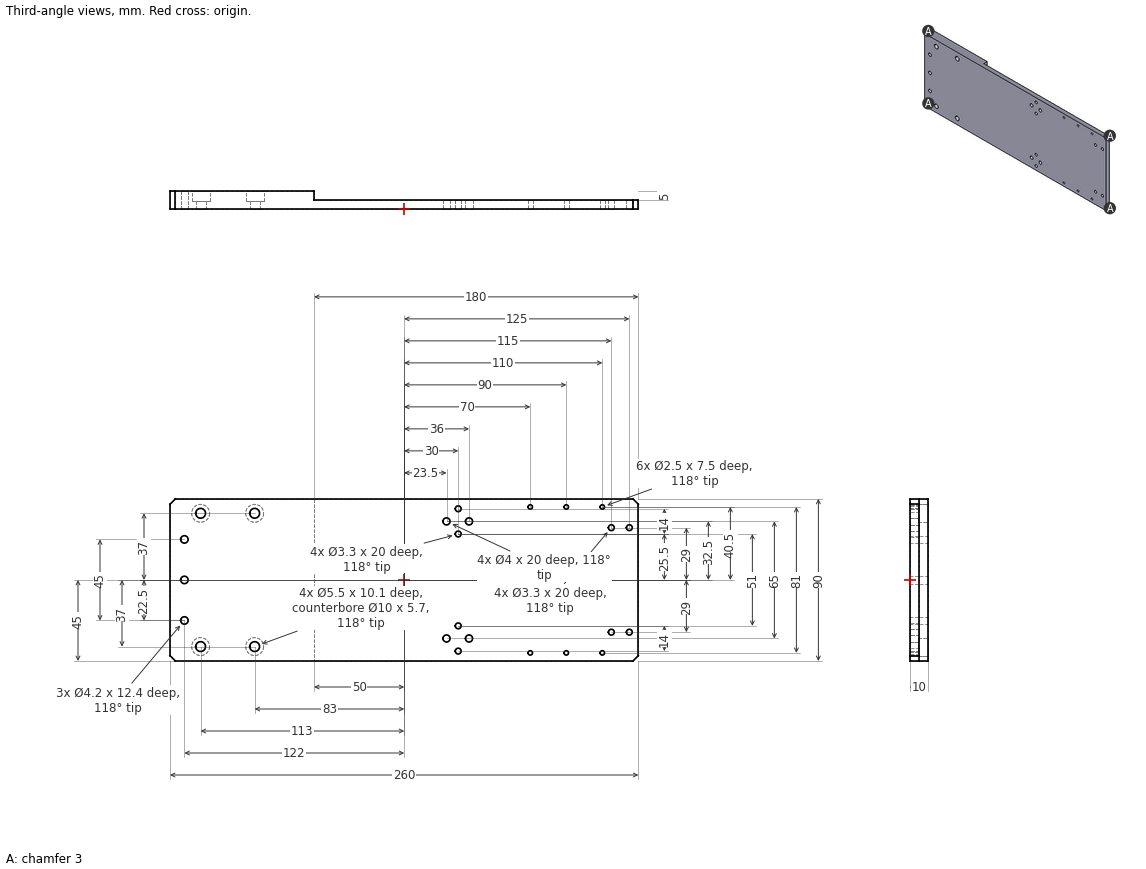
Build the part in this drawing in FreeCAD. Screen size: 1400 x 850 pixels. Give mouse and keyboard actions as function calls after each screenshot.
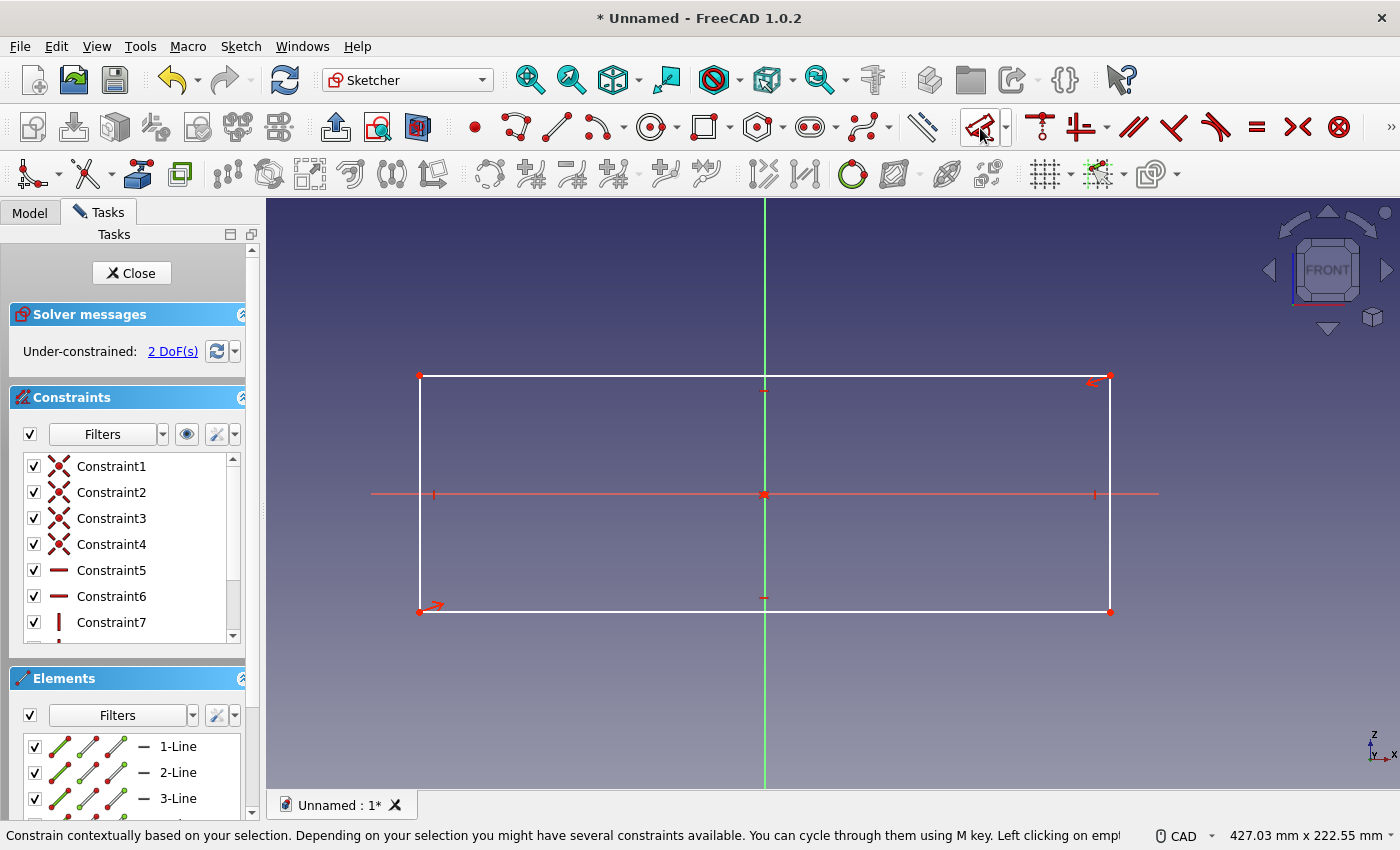
click(1110, 541)
click(1144, 440)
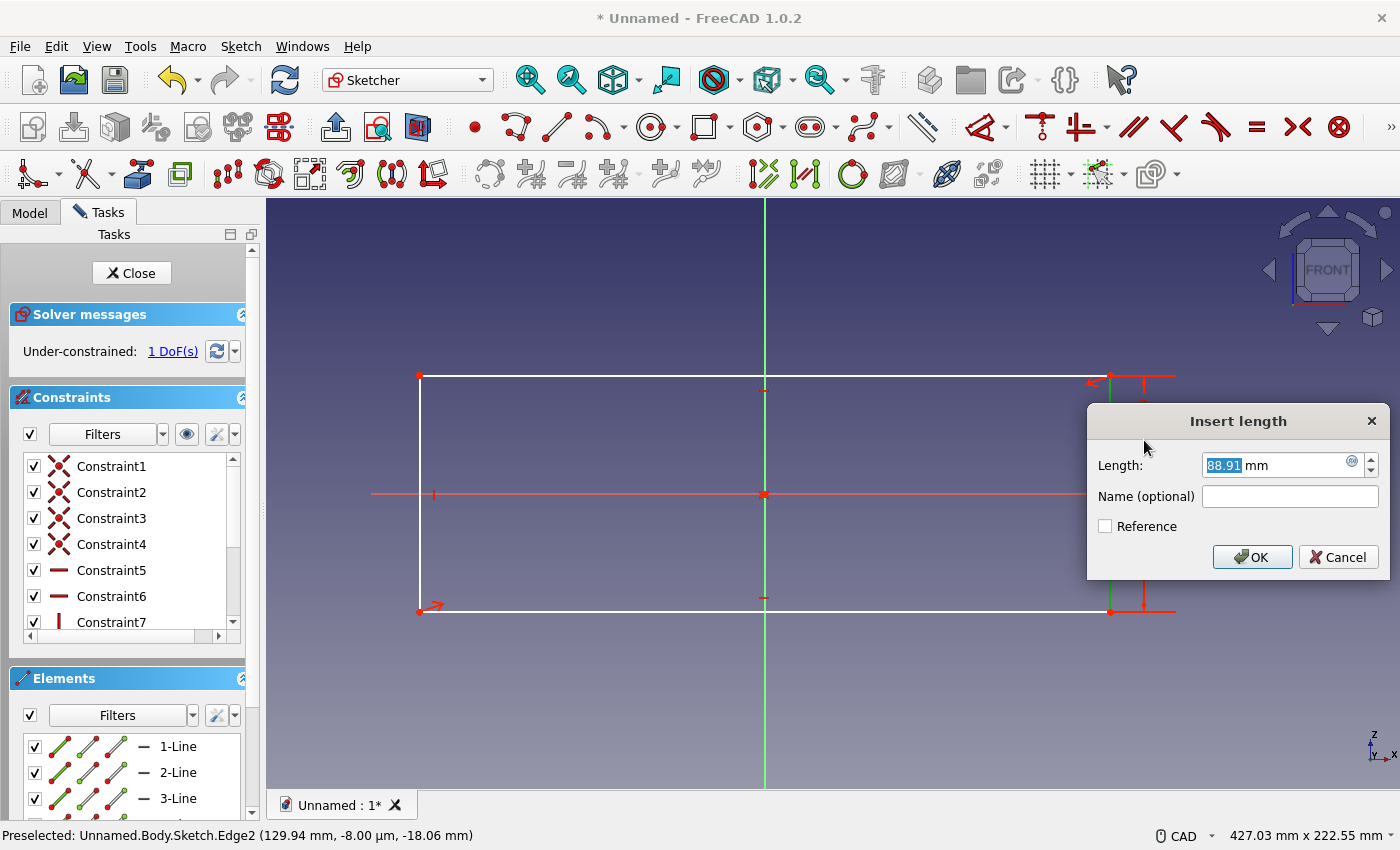
text(90)
key(Return)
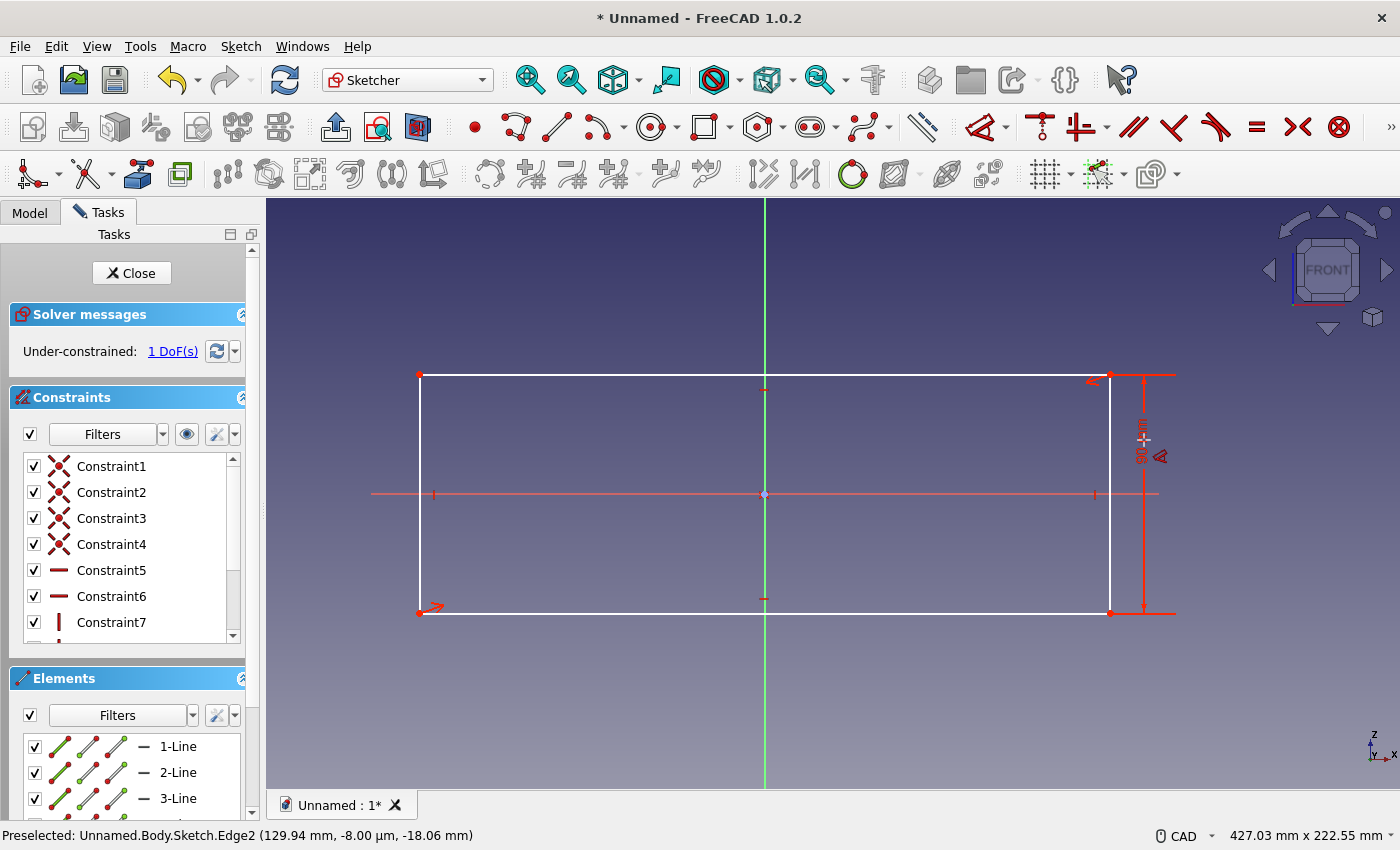
click(627, 614)
click(606, 648)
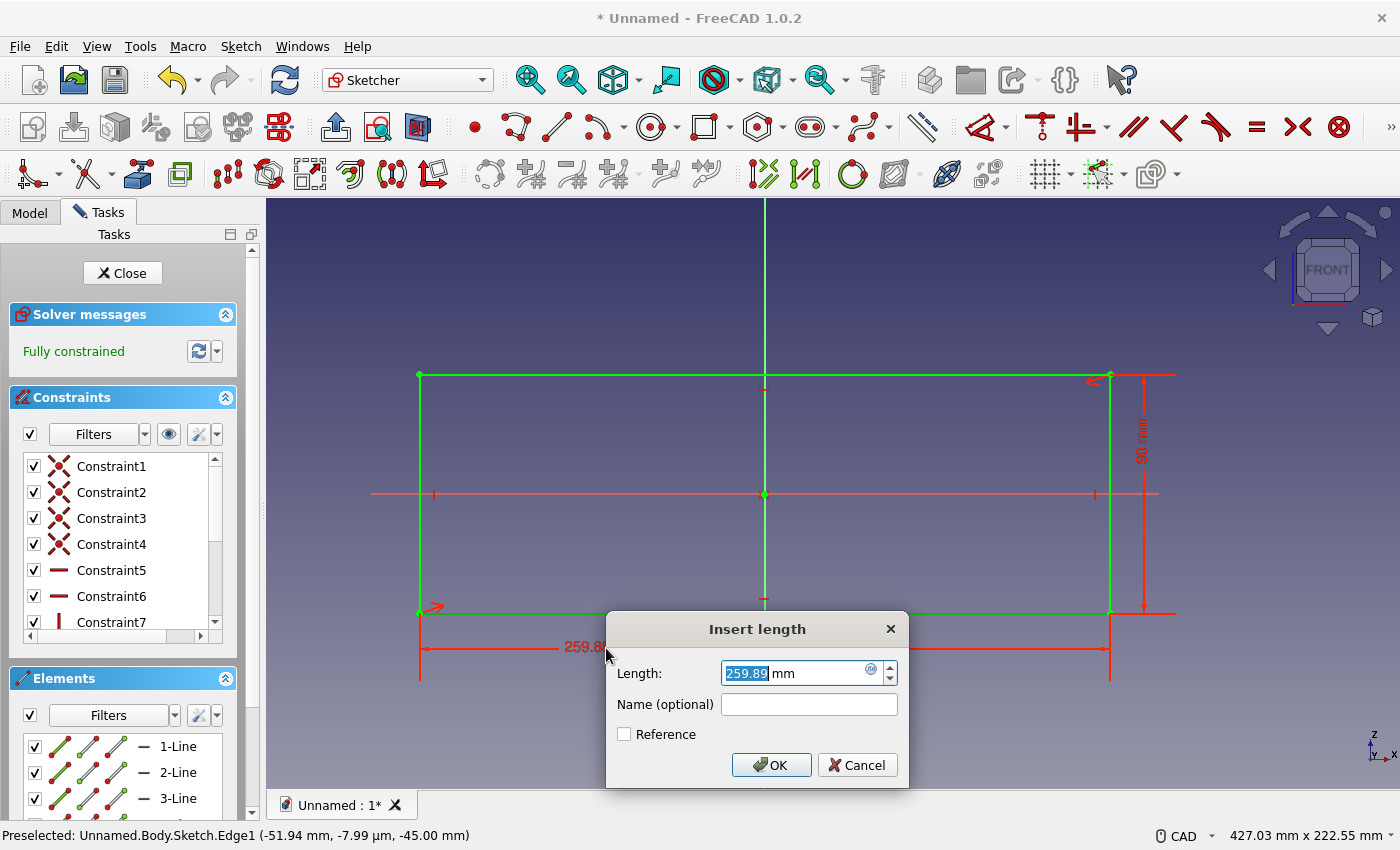
text(260)
key(Return)
key(Escape)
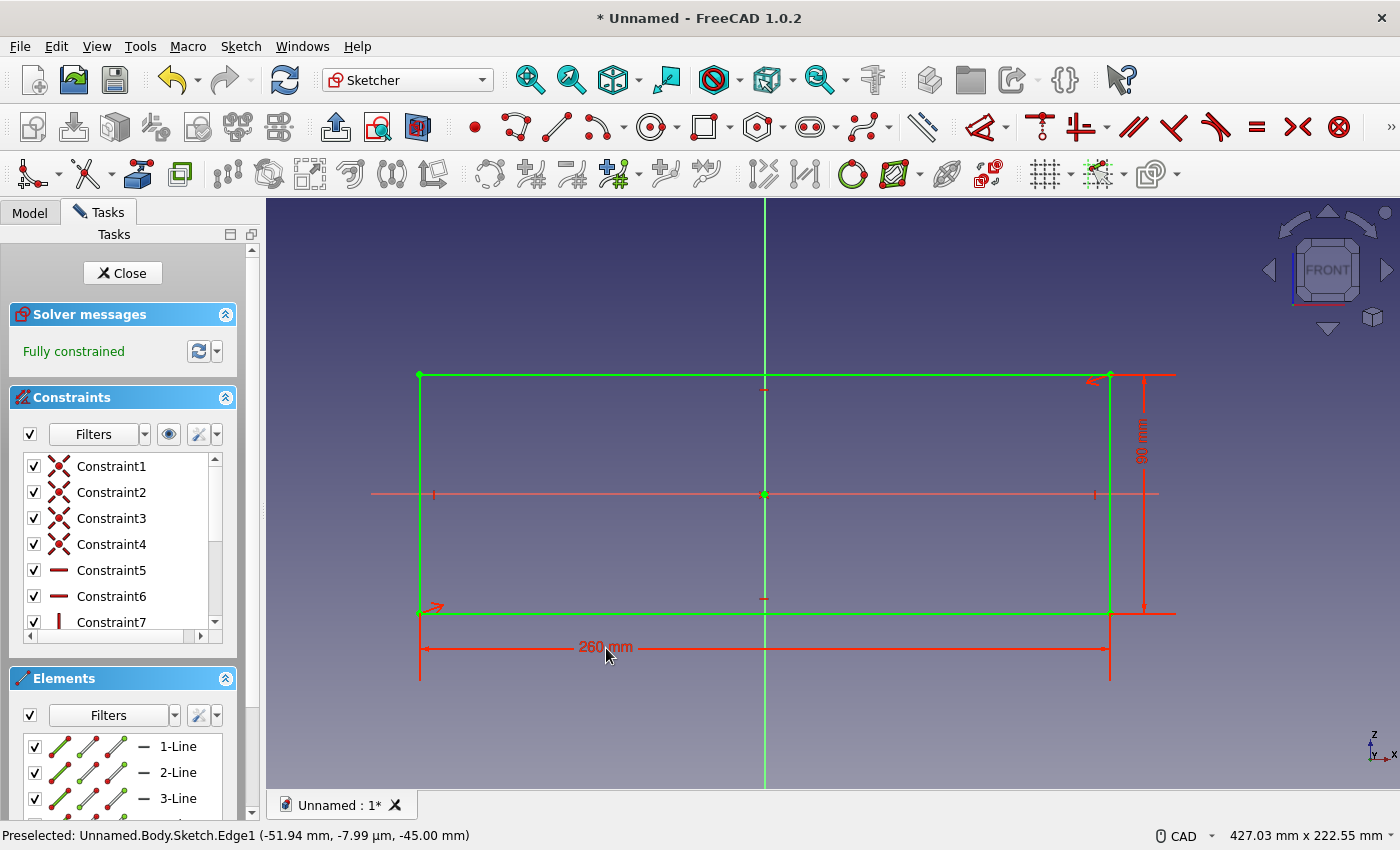
click(123, 273)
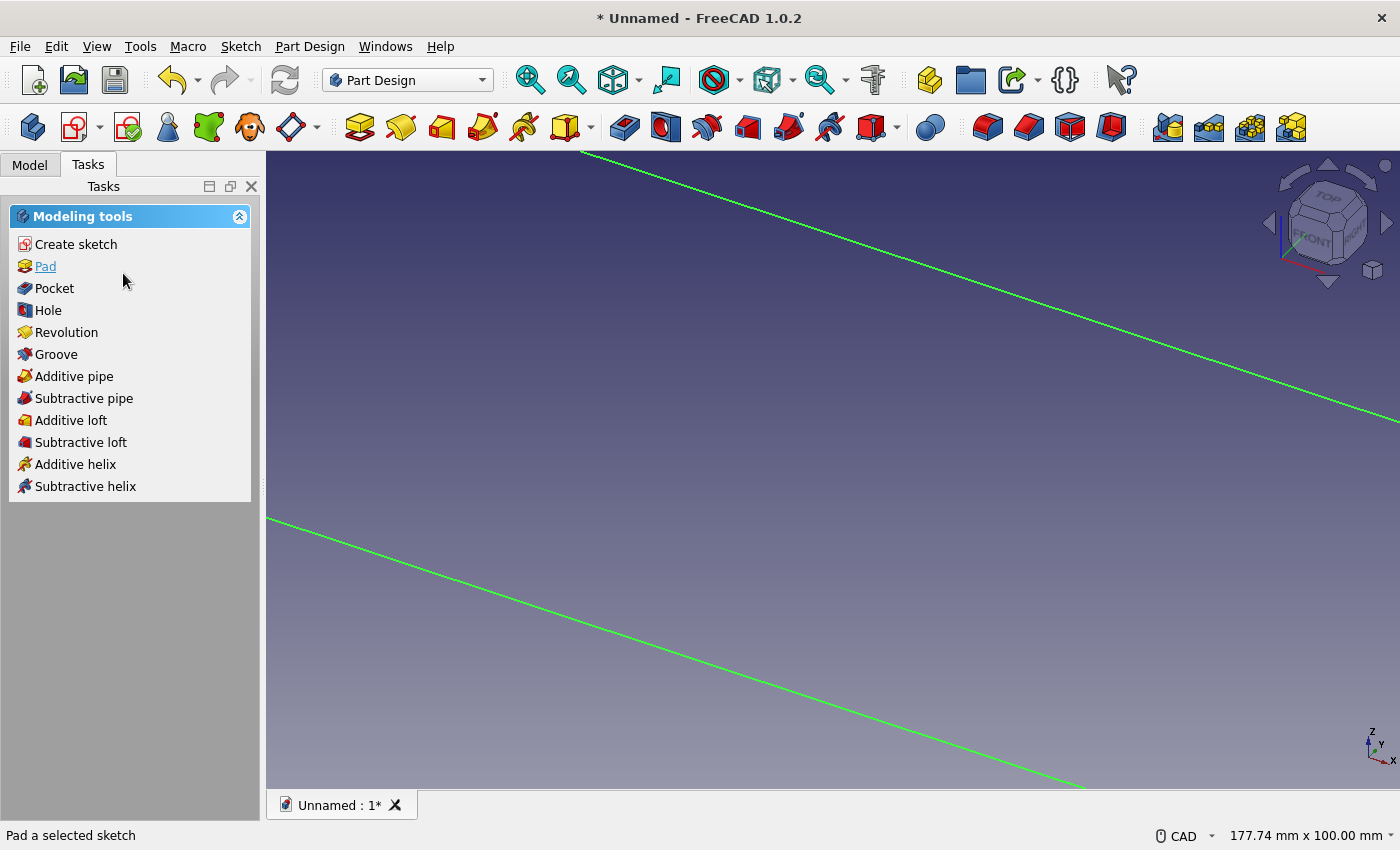
click(360, 128)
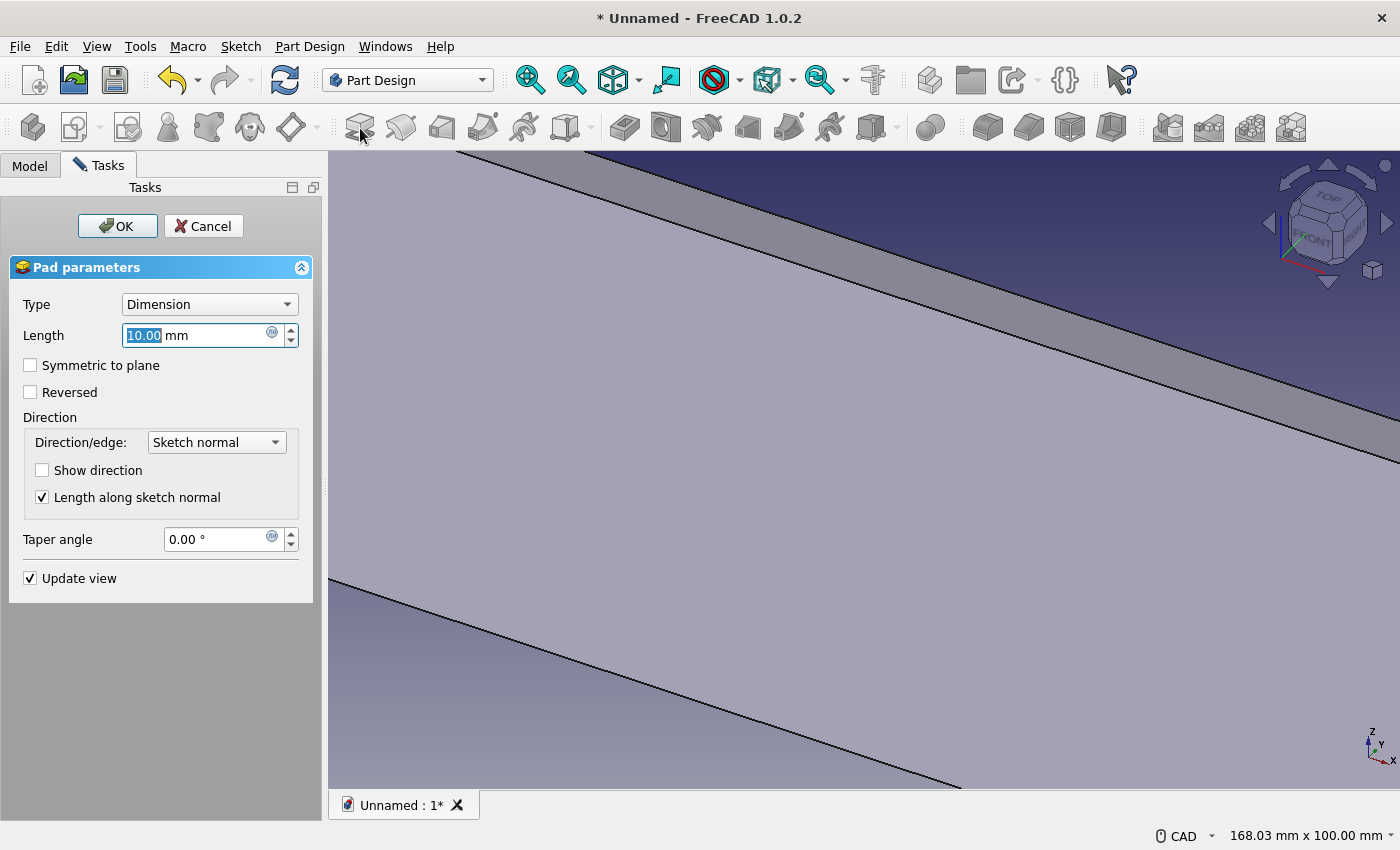
text(10)
key(Tab)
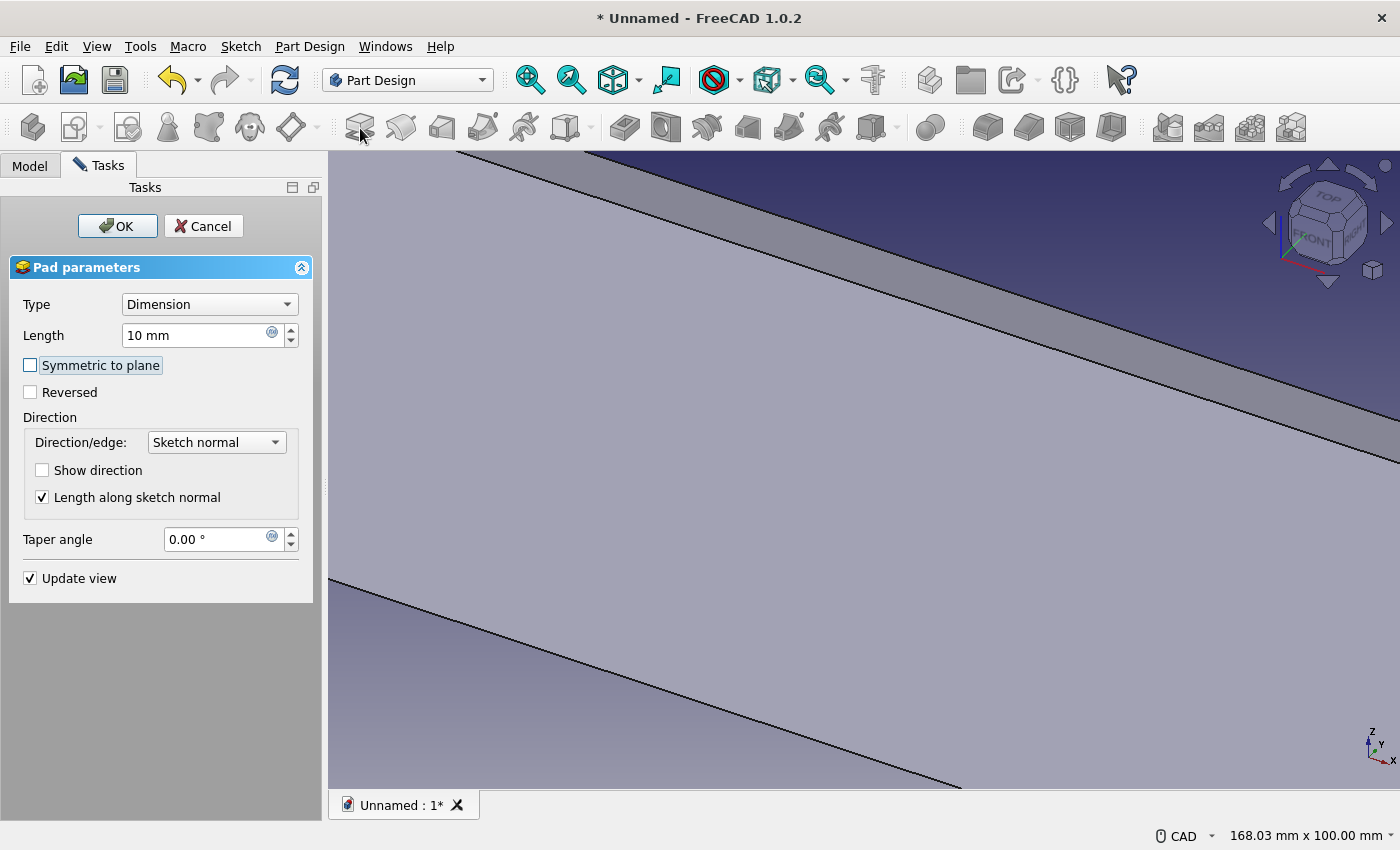
click(31, 392)